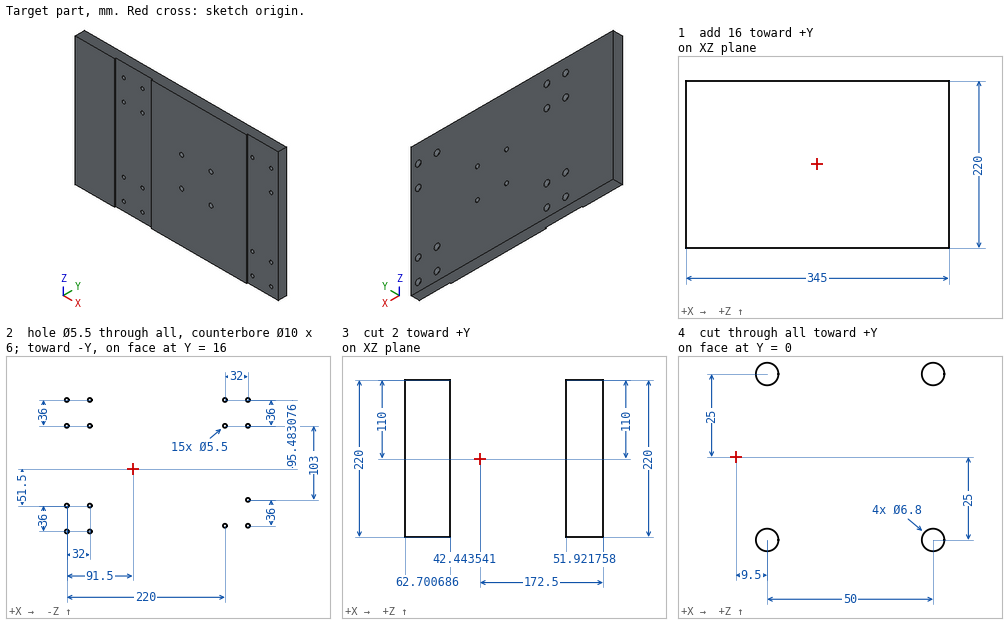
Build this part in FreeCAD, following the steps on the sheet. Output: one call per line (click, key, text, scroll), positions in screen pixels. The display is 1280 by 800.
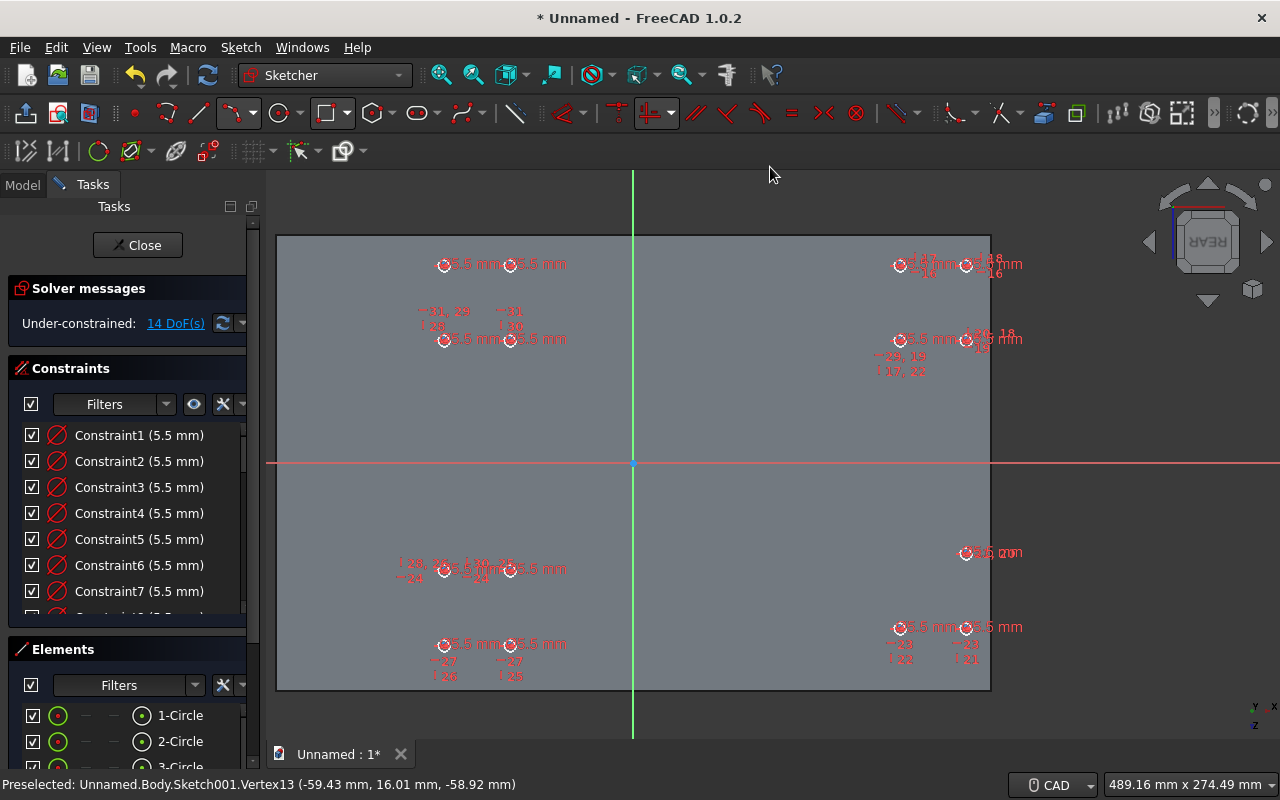
click(510, 341)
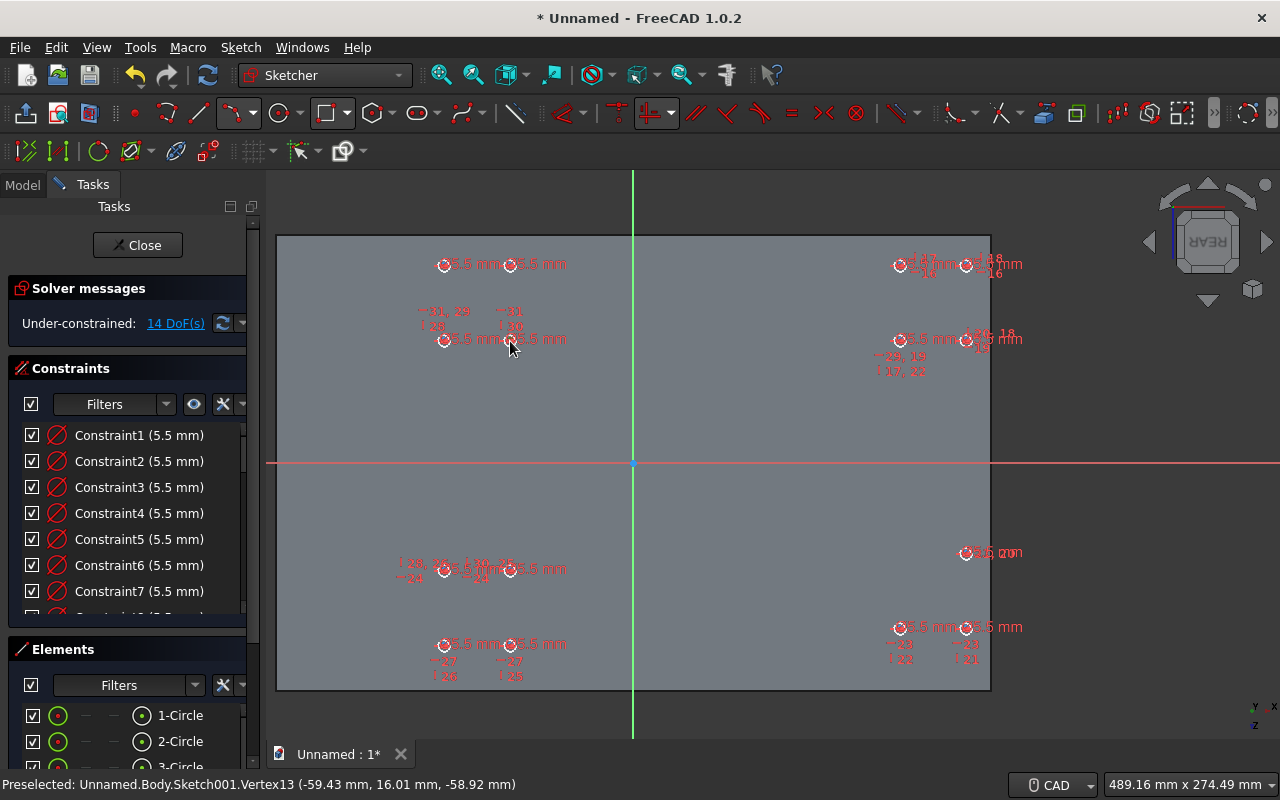
click(510, 266)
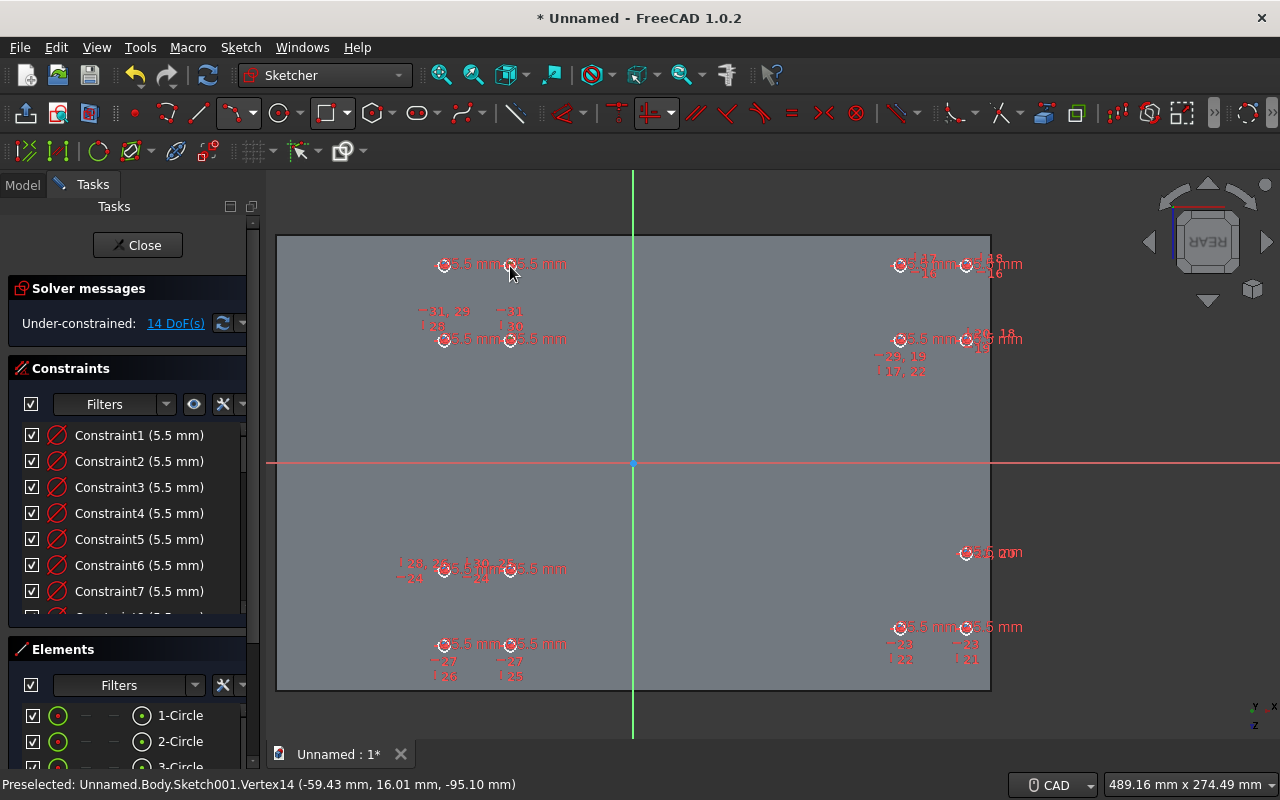
key(v)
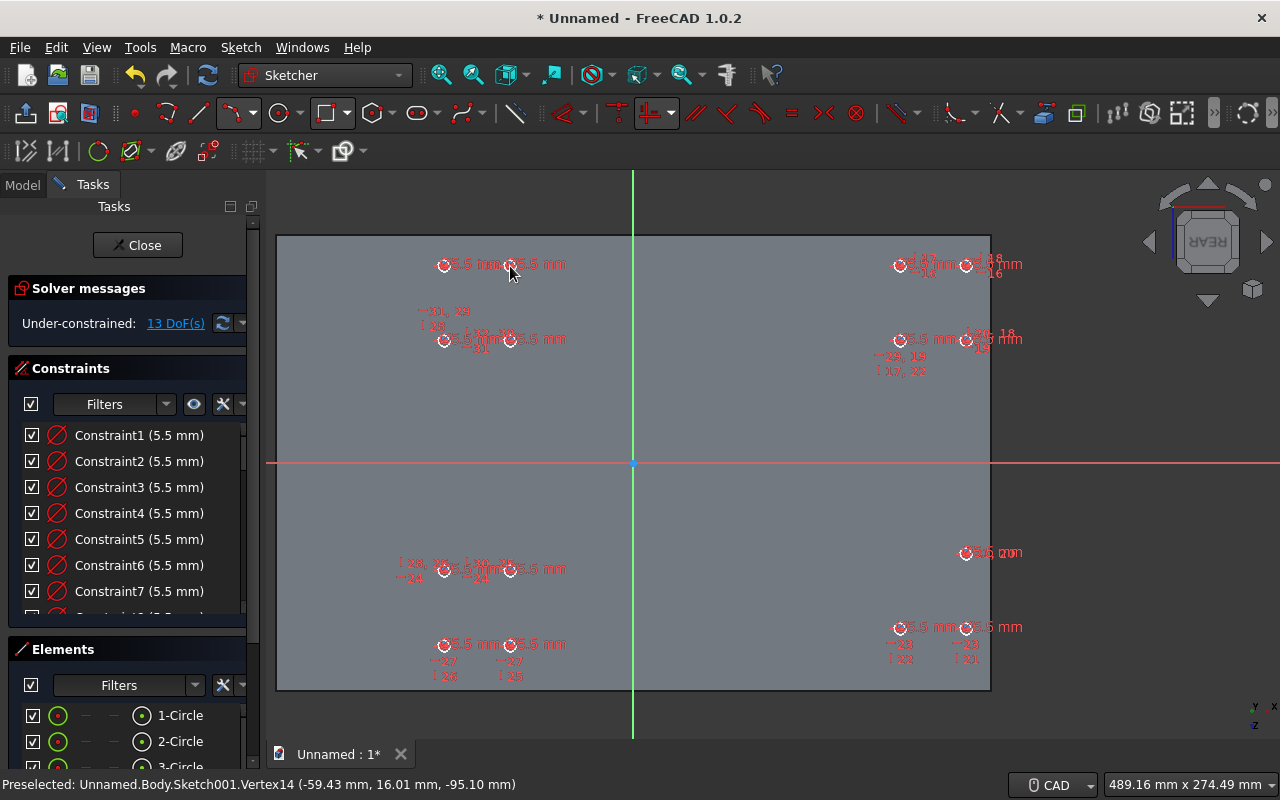
click(444, 341)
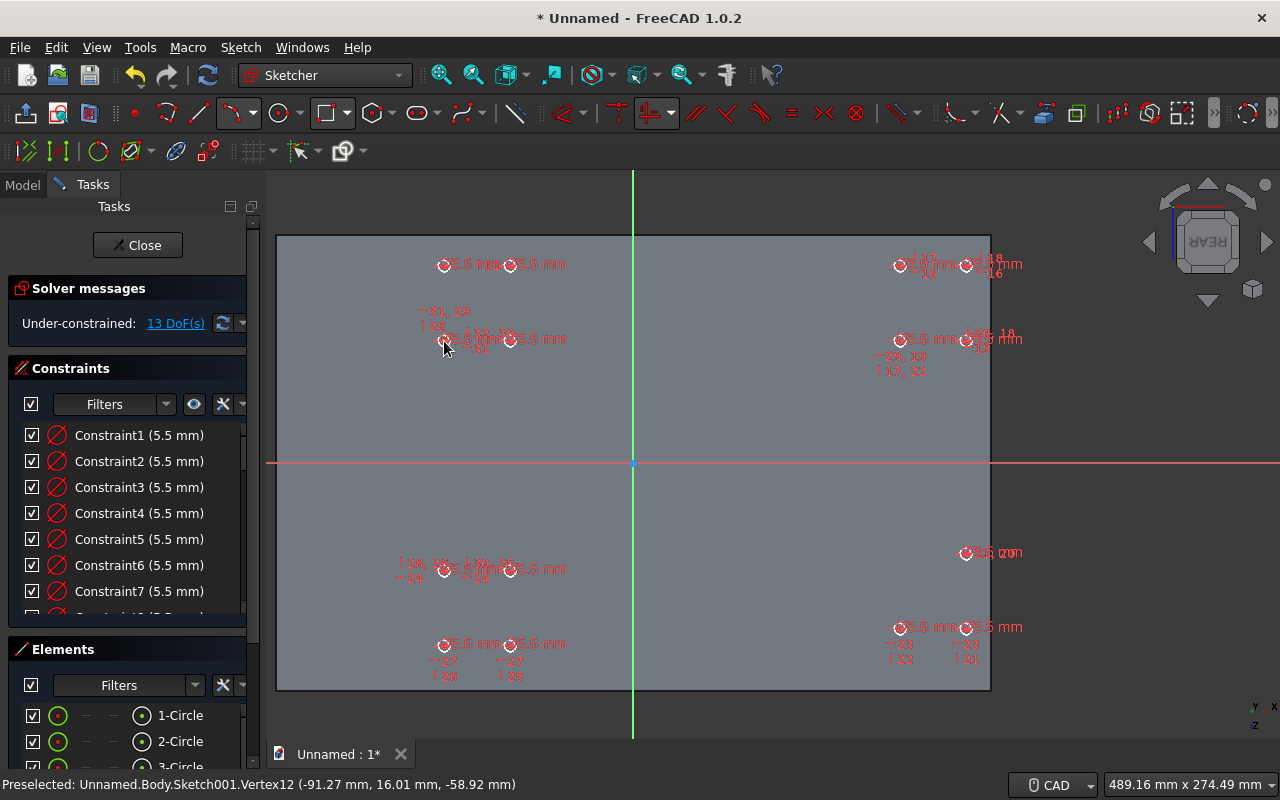
click(444, 266)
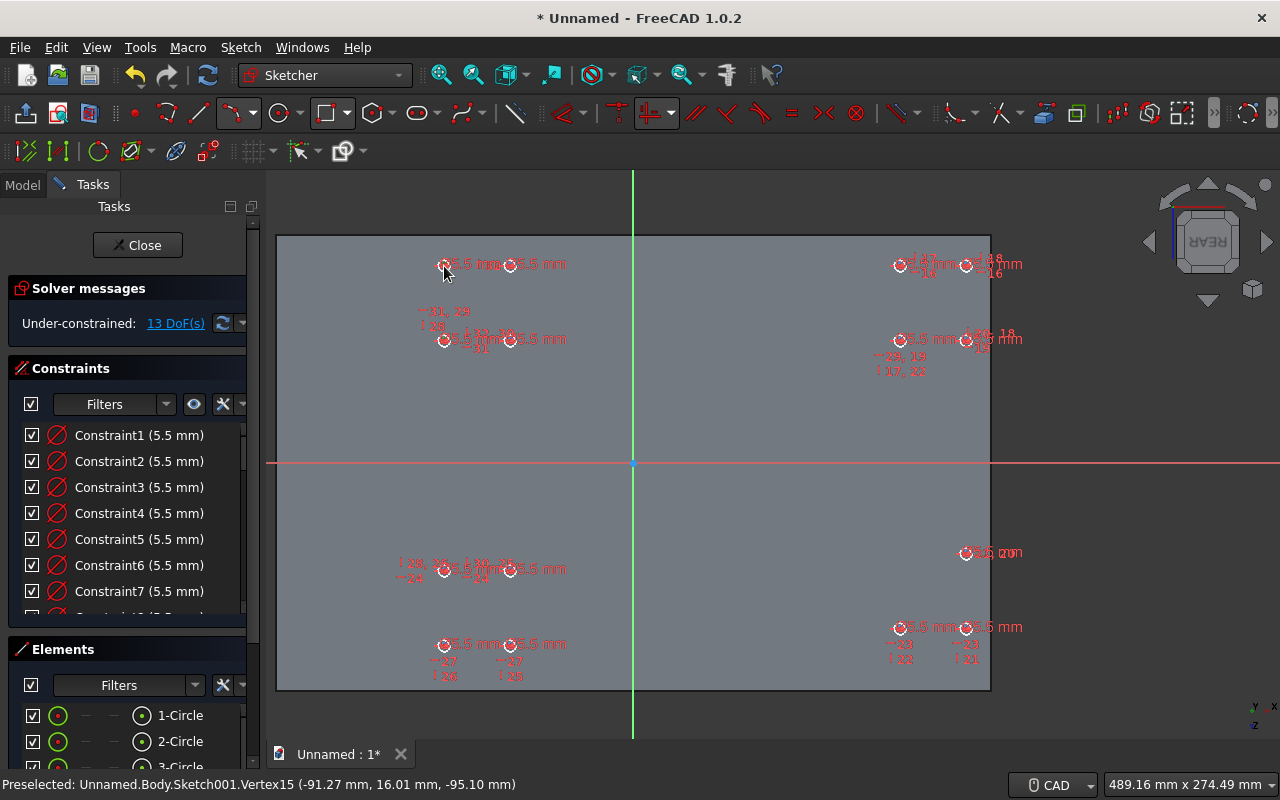
click(674, 114)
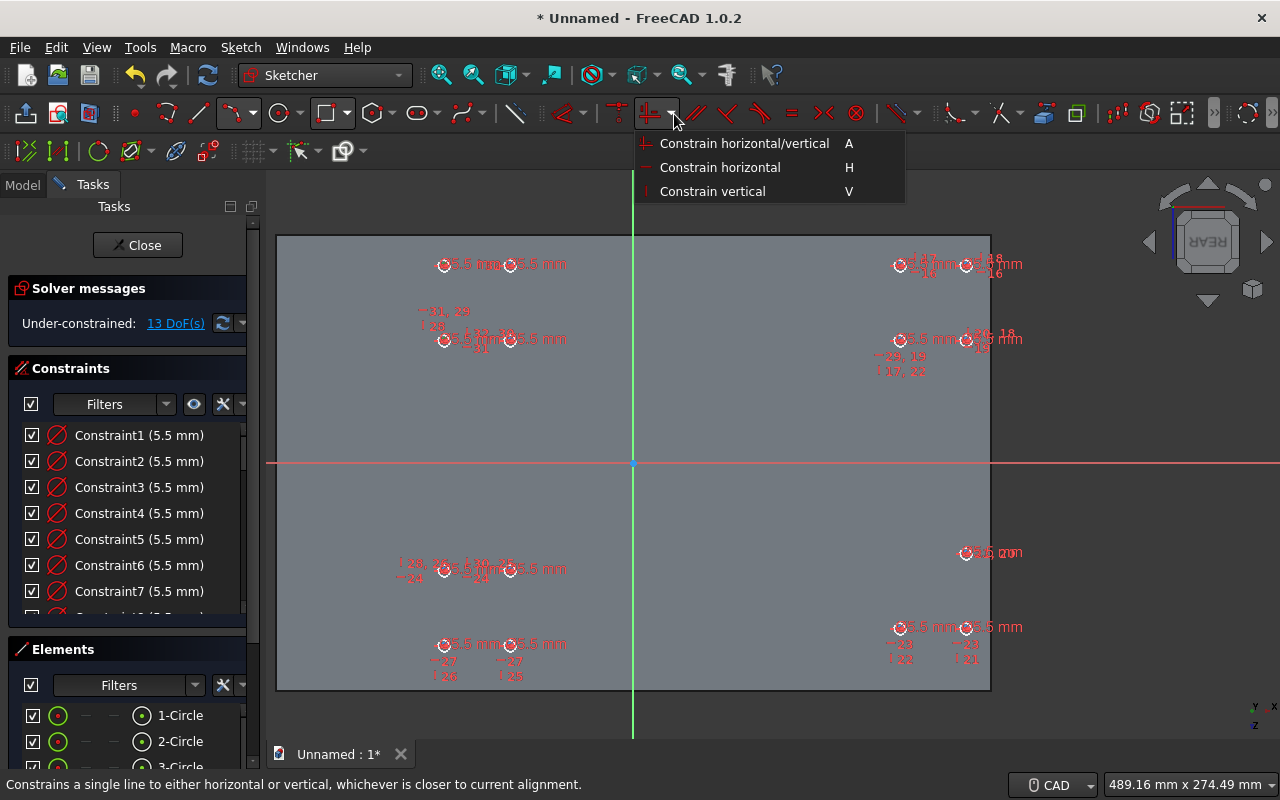
click(770, 191)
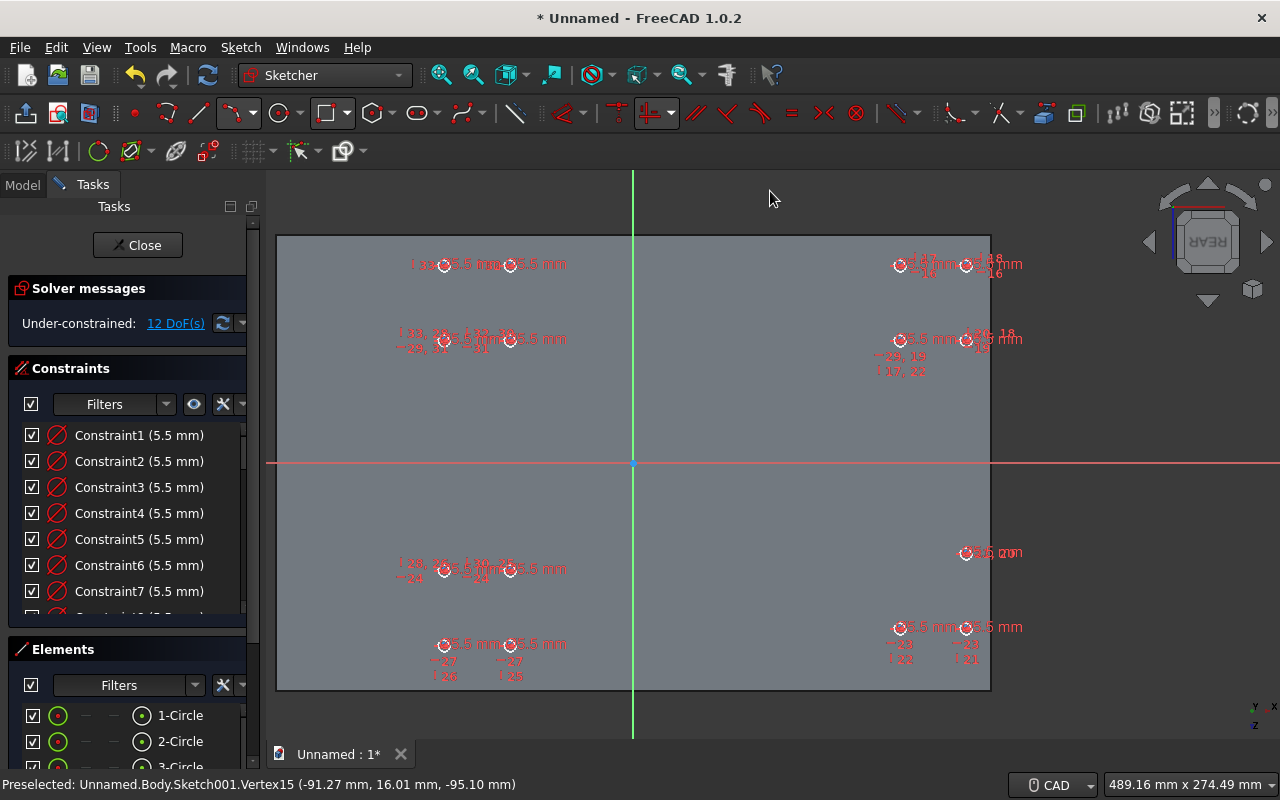
click(510, 266)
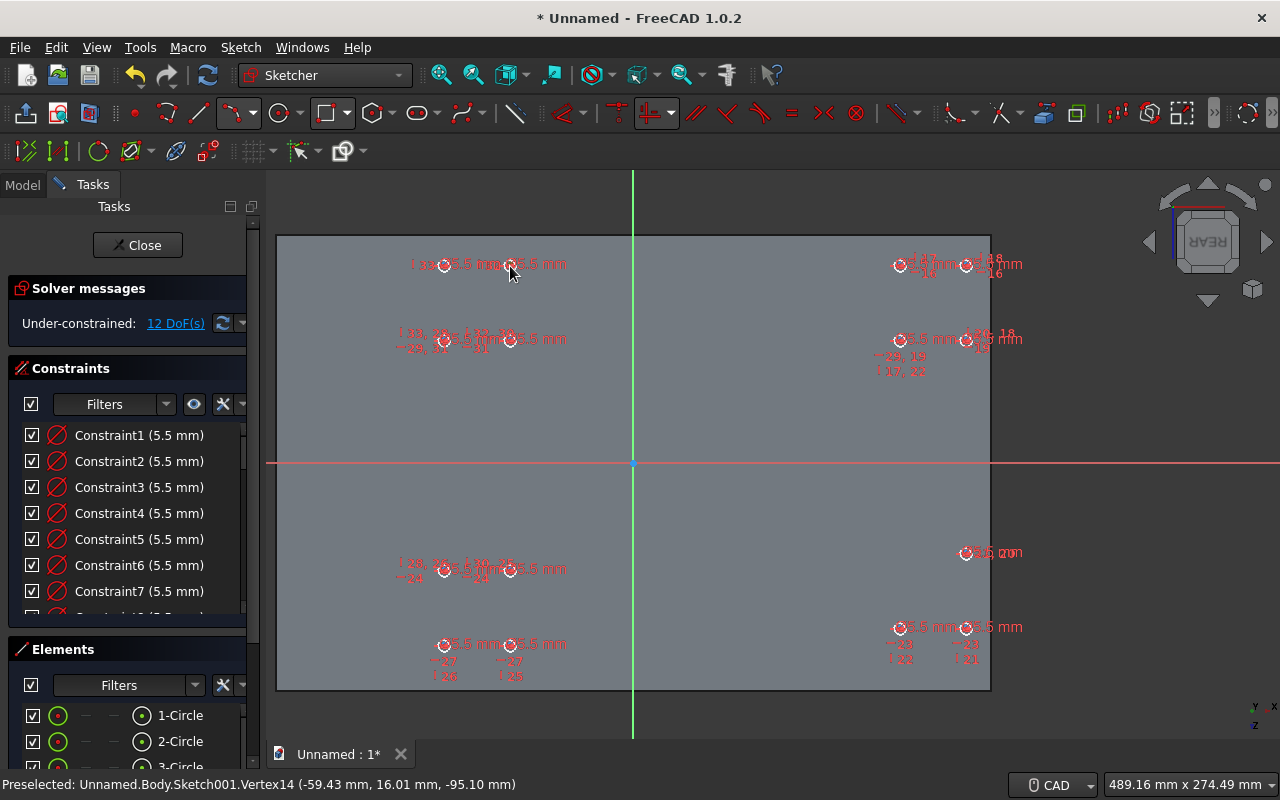
click(444, 266)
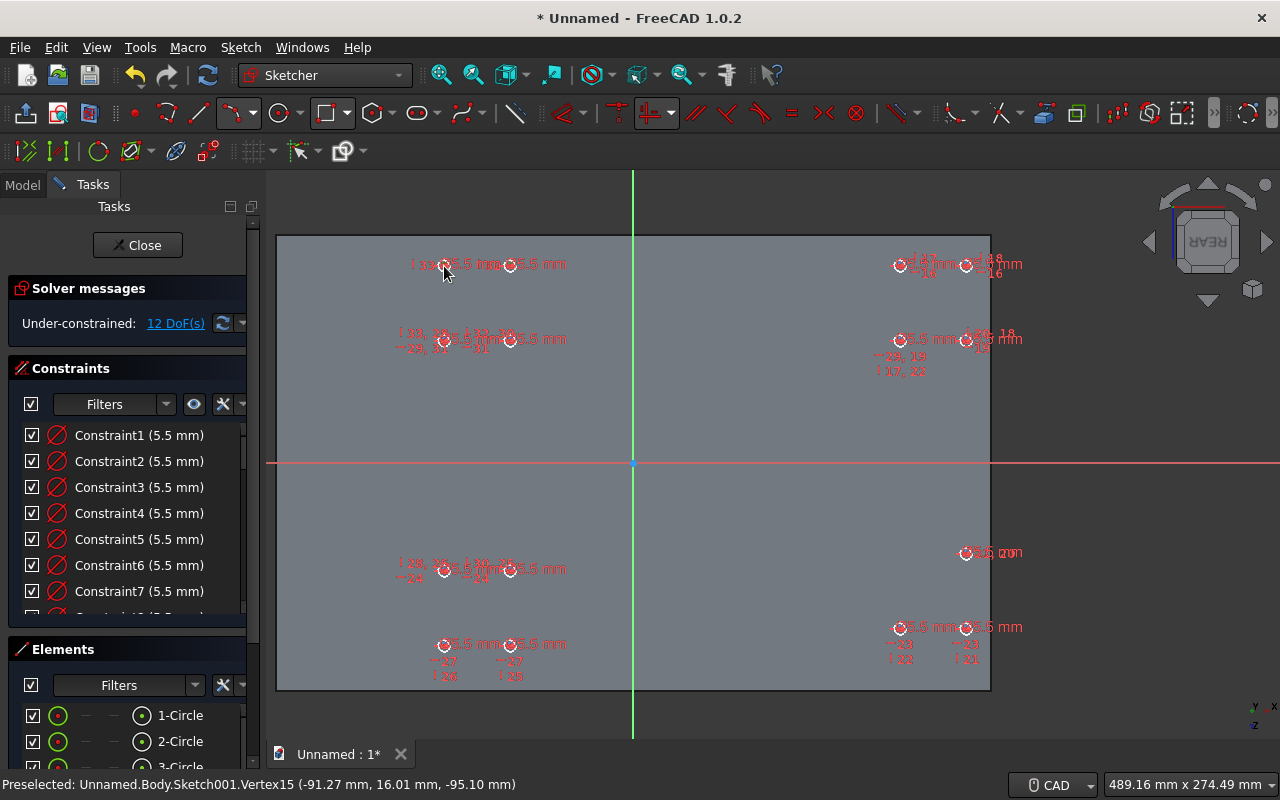
key(h)